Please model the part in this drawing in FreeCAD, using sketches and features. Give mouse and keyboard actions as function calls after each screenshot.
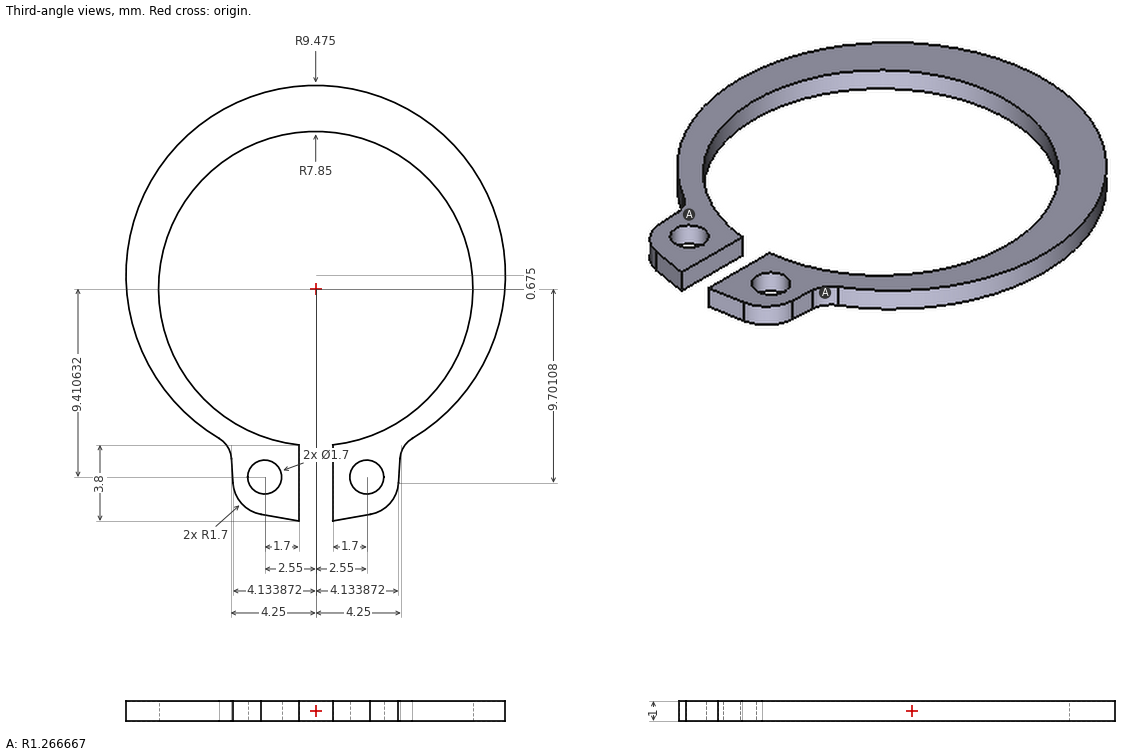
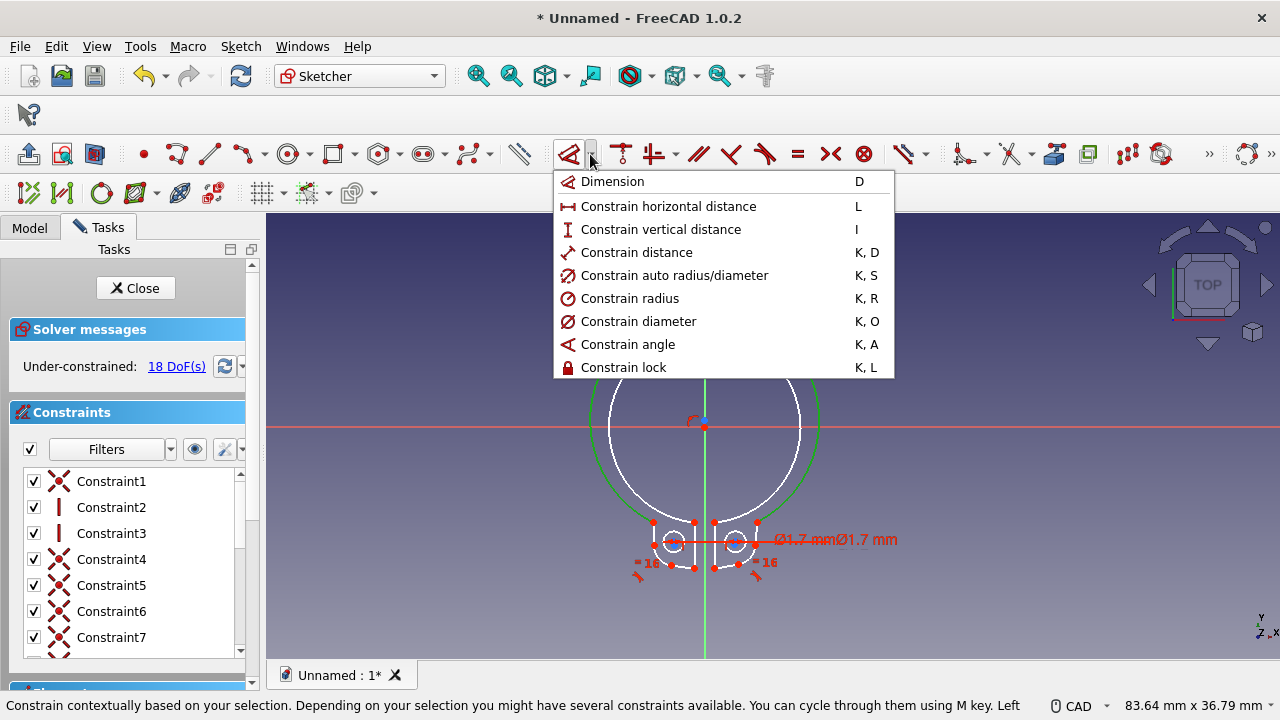
click(724, 298)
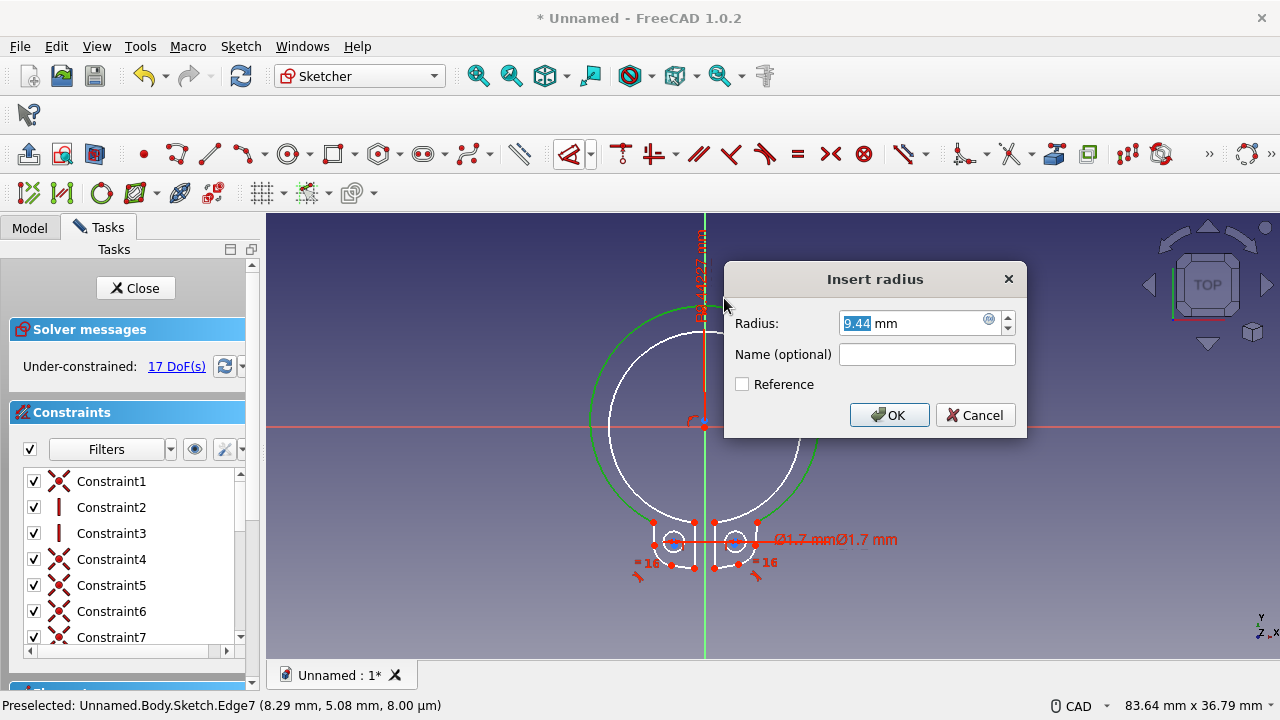
text(9.475)
key(Return)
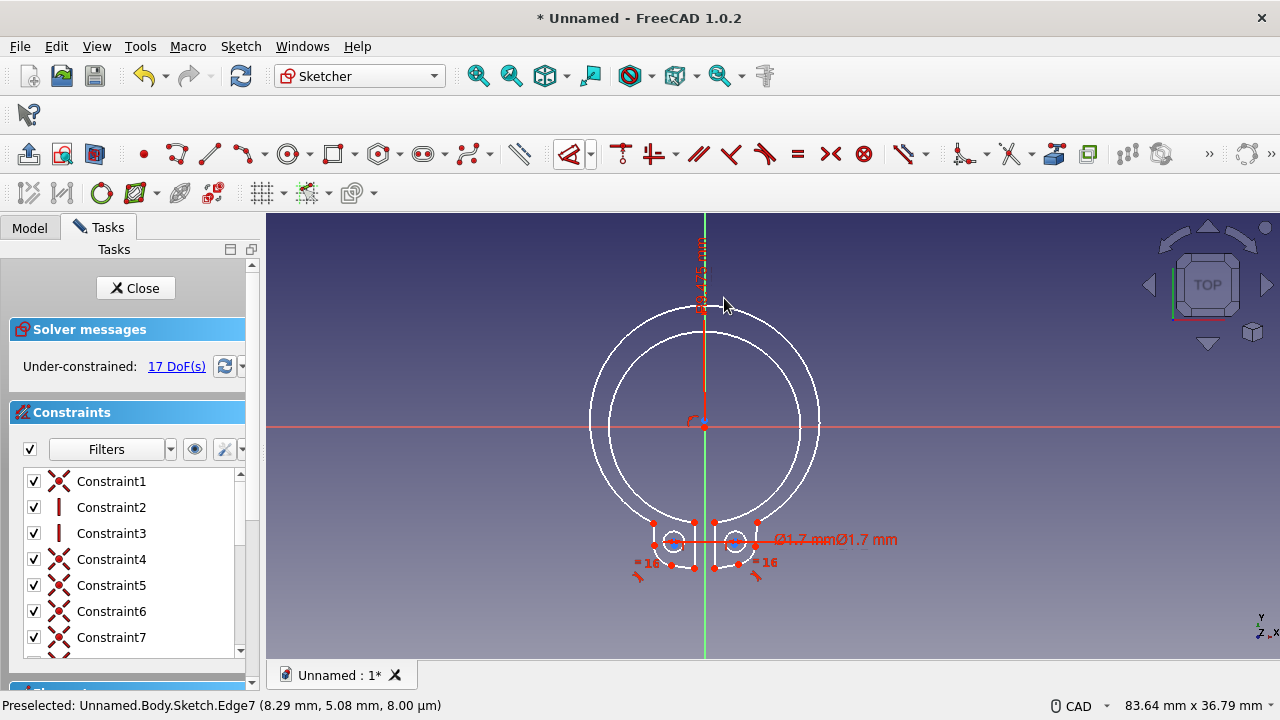
scroll(659, 559, up, 4)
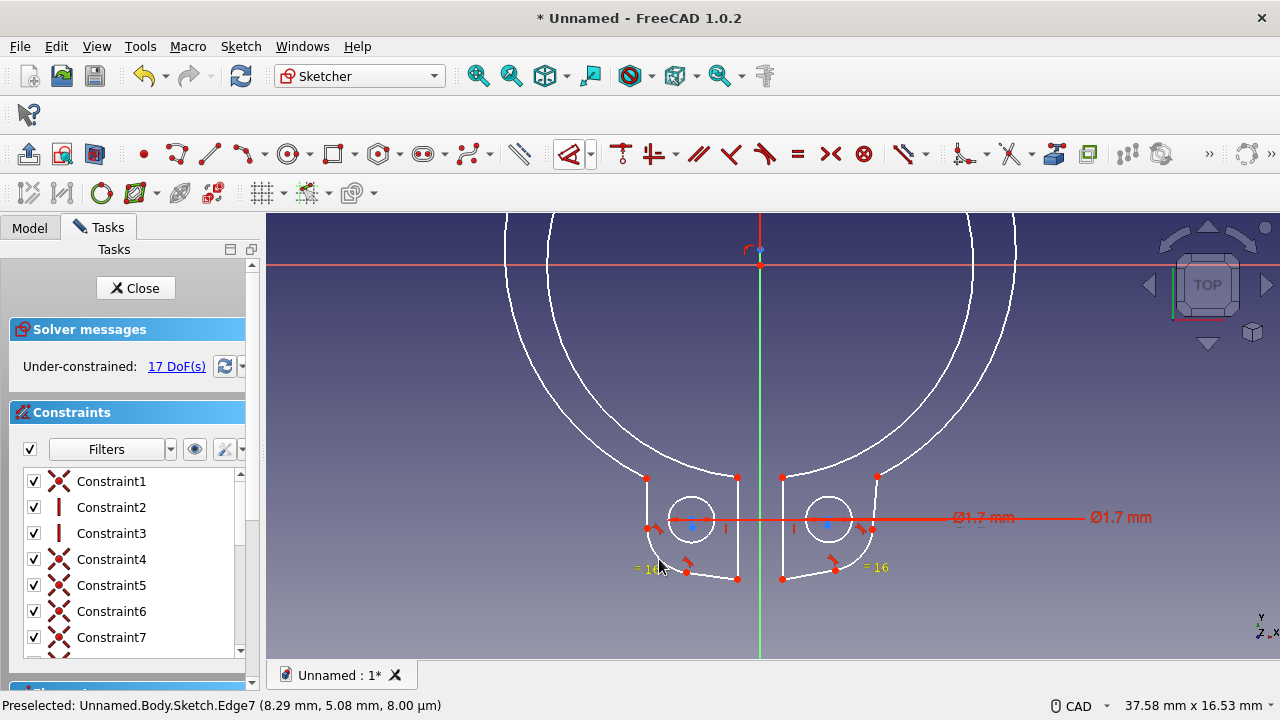
click(659, 558)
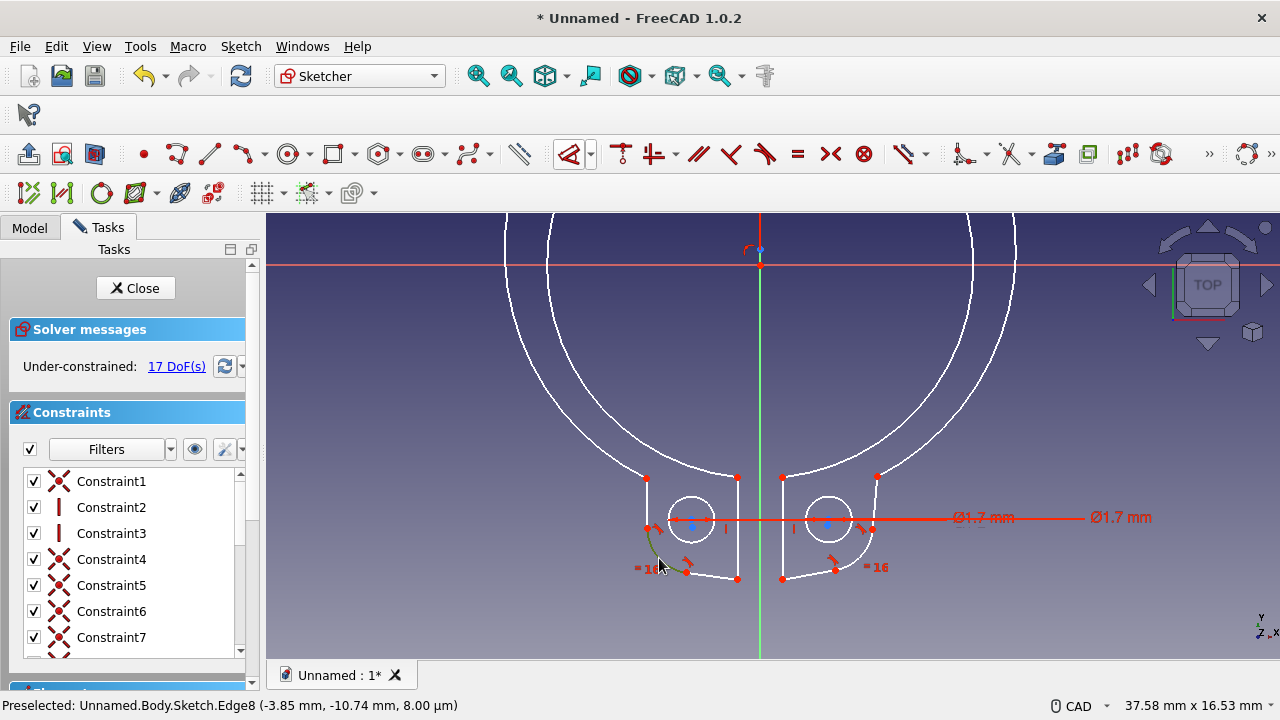
click(590, 154)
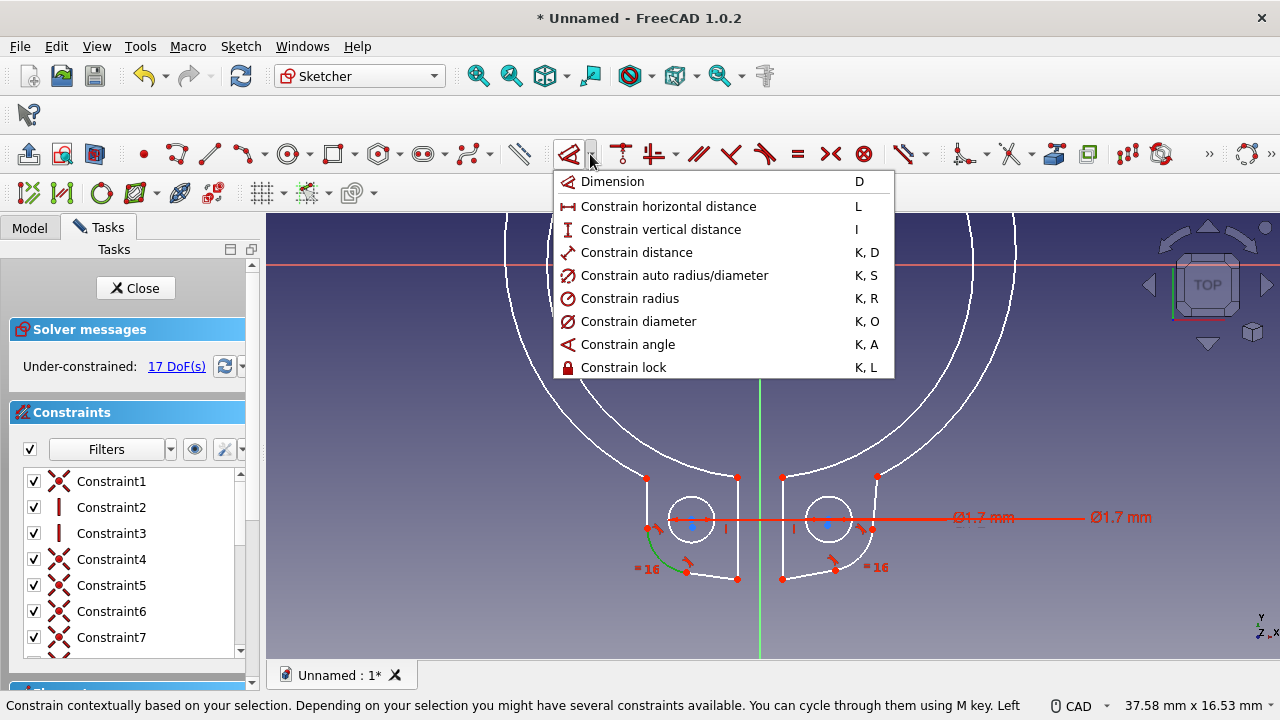
click(724, 298)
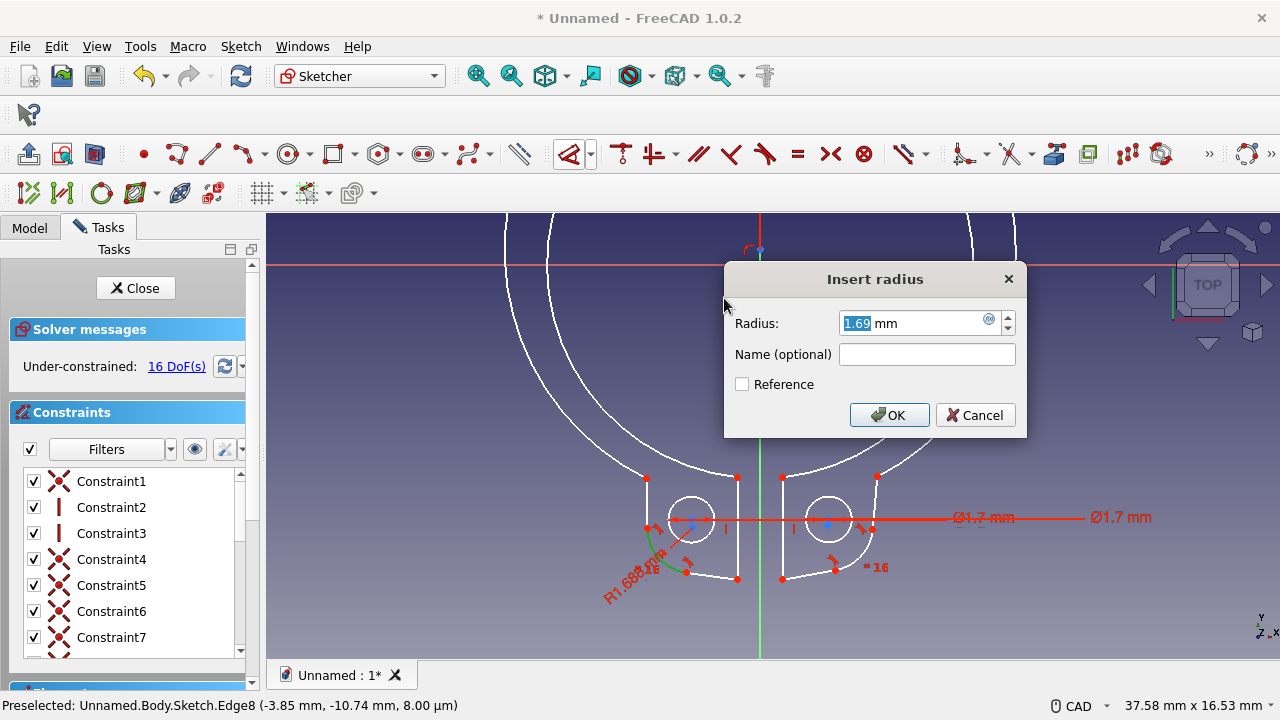
text(1.7)
key(Return)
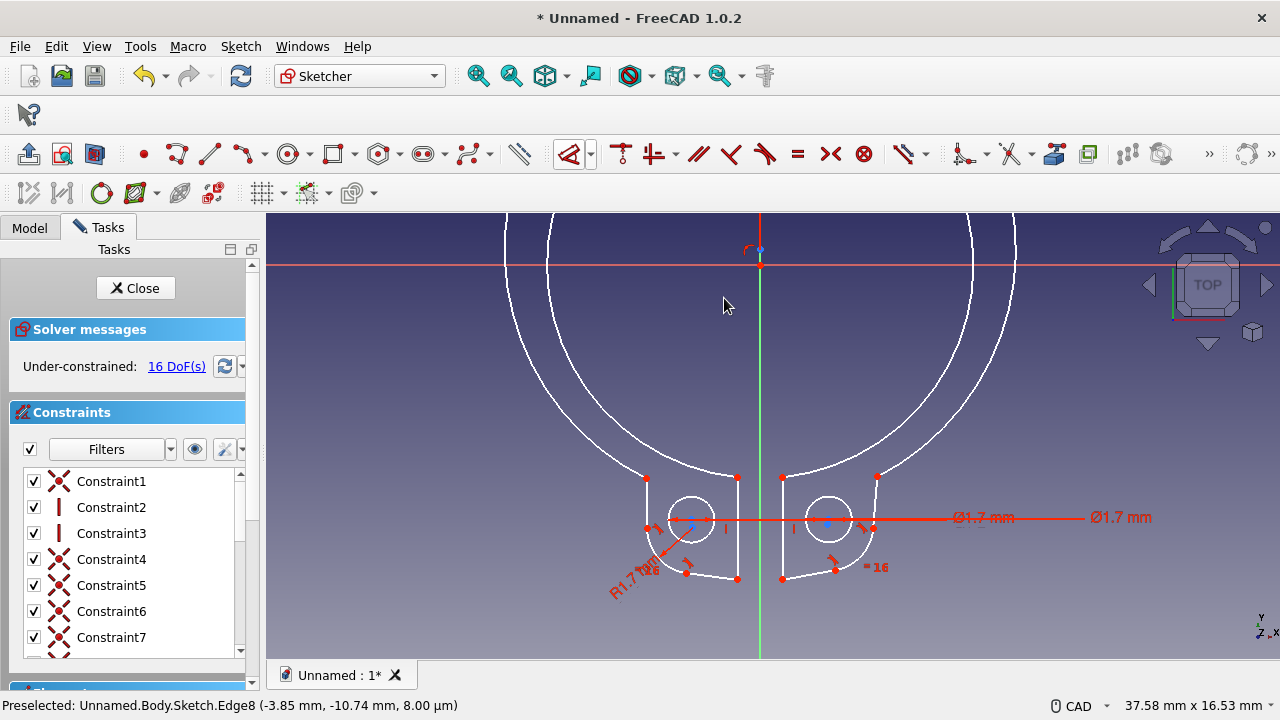
click(967, 318)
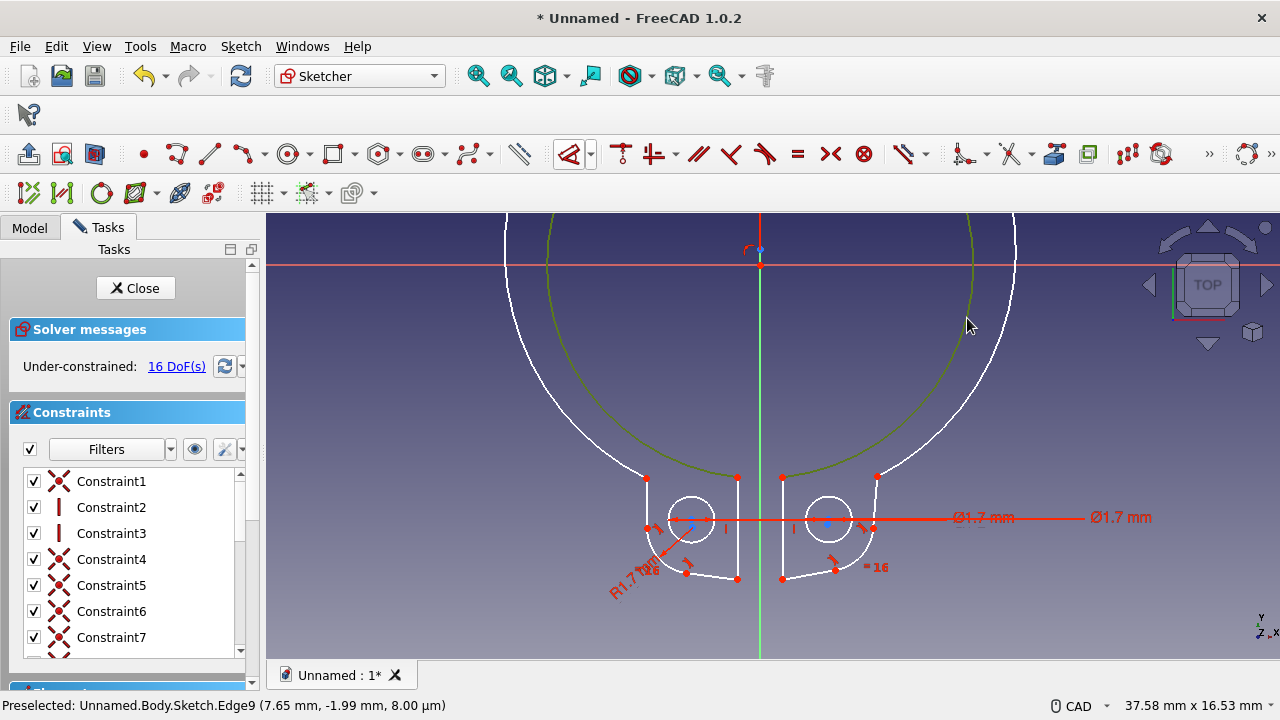
key(k)
key(r)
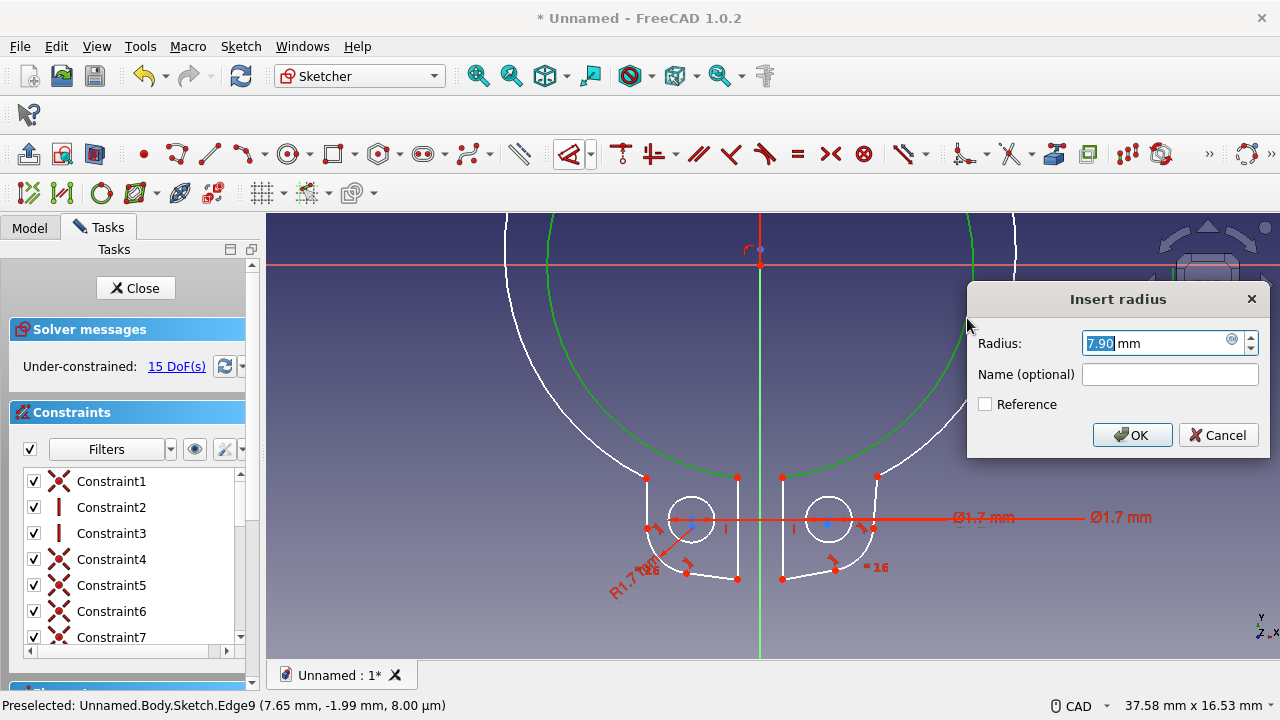
text(7.85)
key(Return)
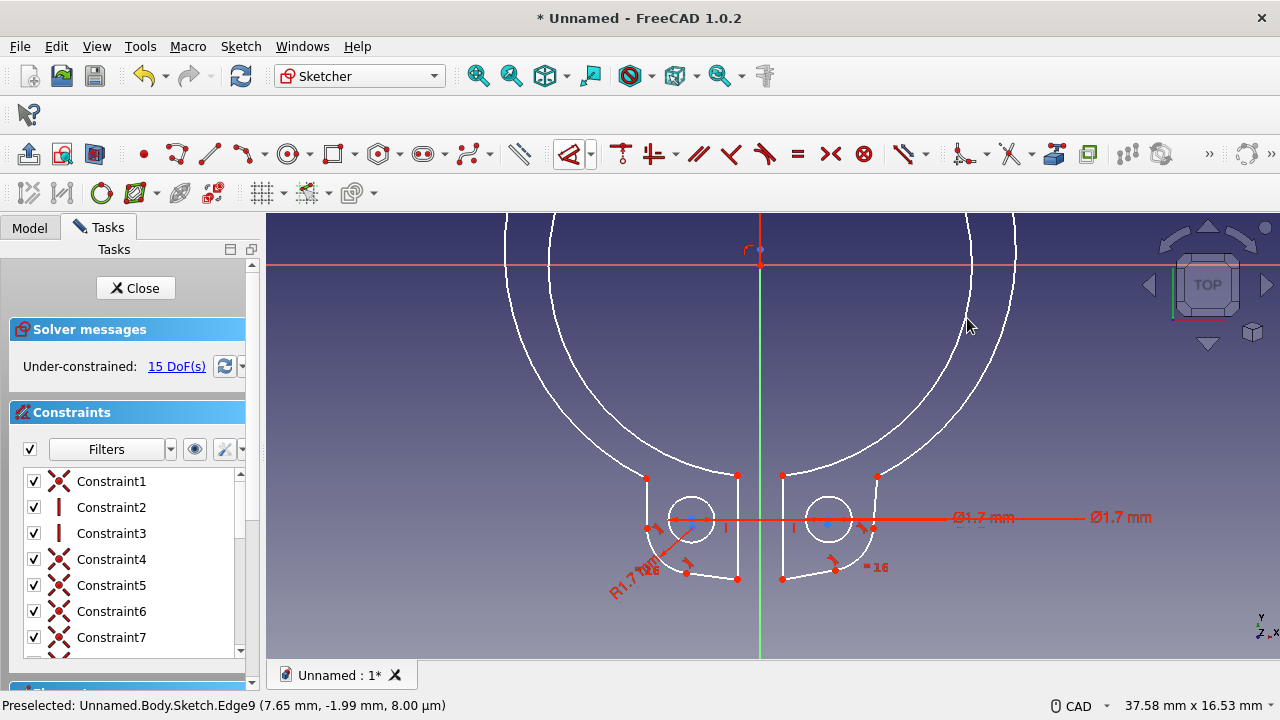
click(738, 549)